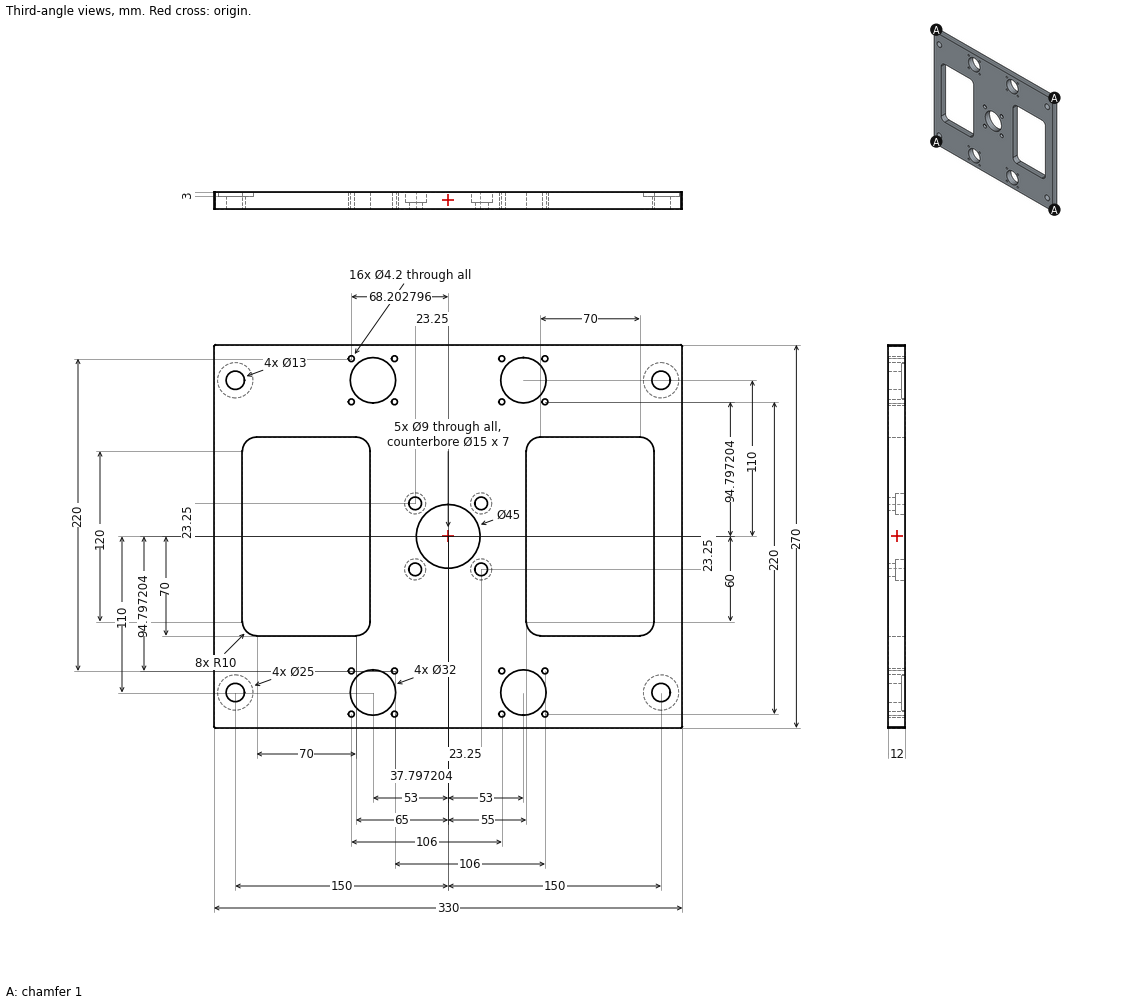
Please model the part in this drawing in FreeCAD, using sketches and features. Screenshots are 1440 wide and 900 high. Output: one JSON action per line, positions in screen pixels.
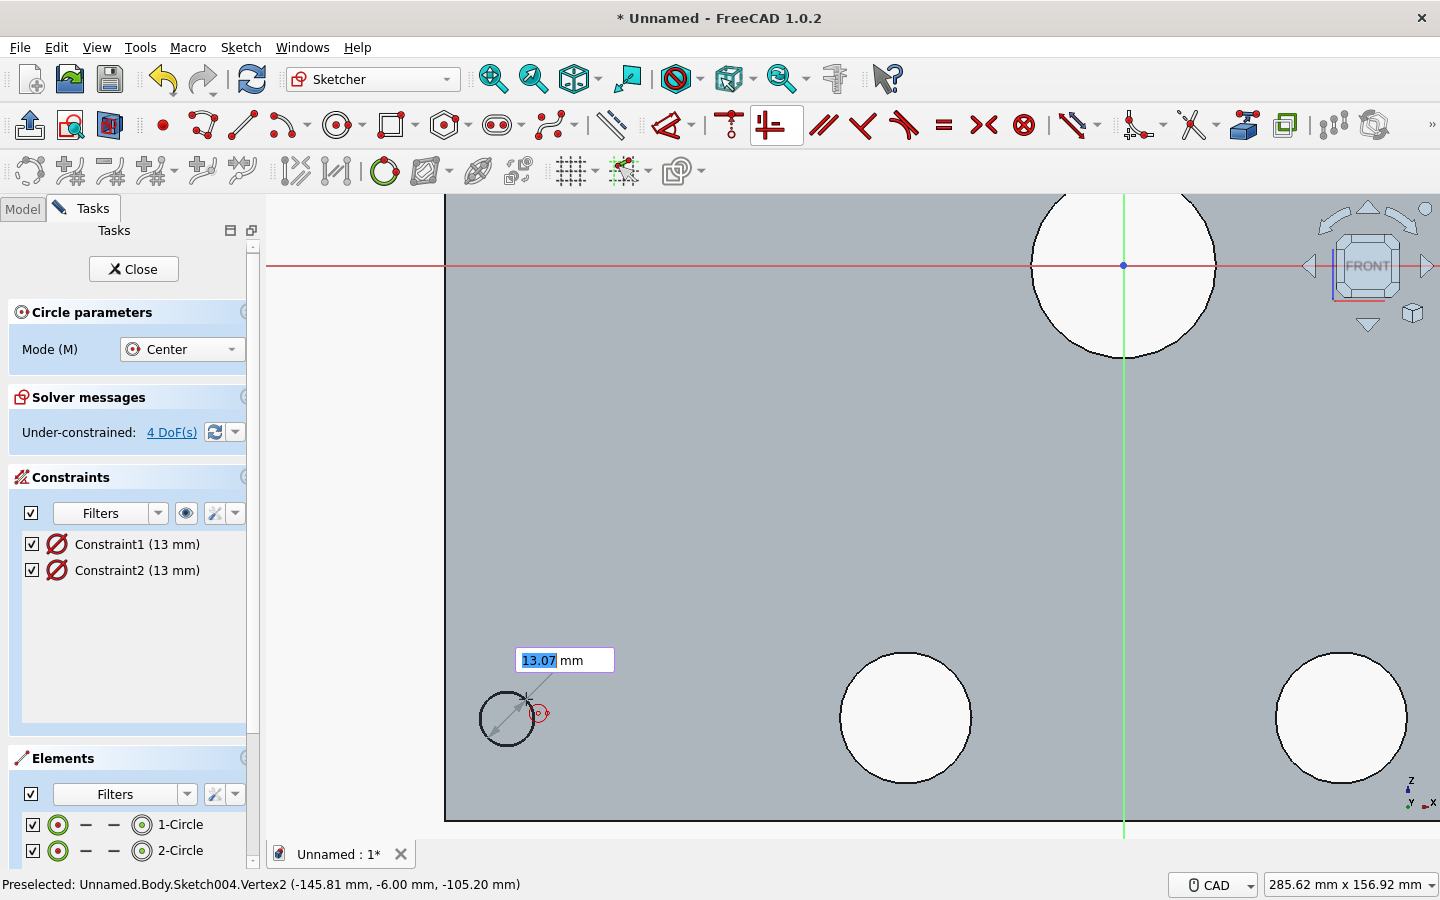
{"action": "type", "text": "13"}
{"action": "key", "text": "Return"}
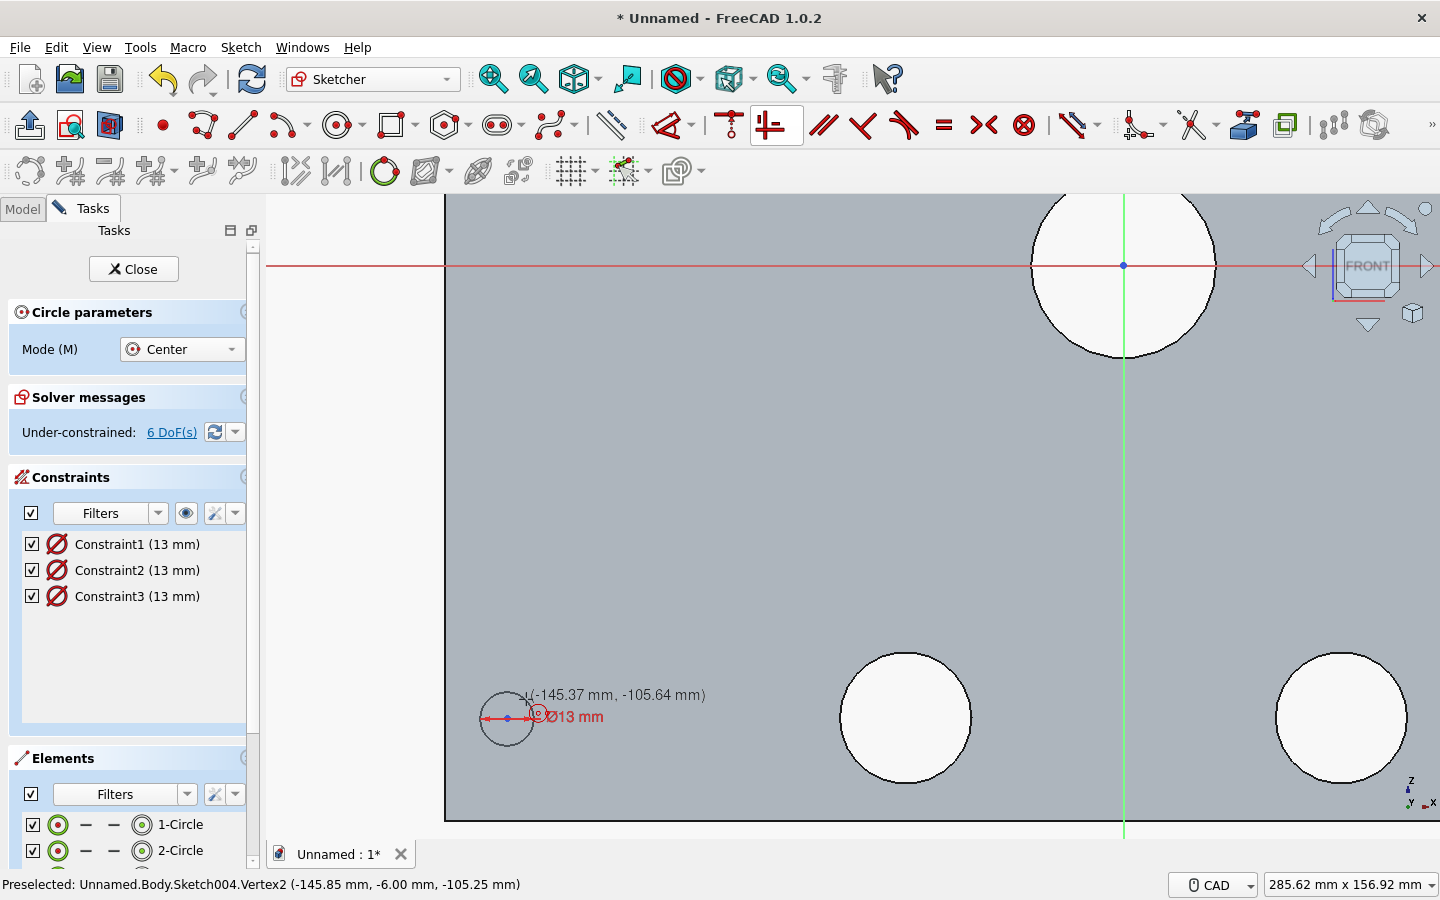
{"action": "scroll", "coordinate": [508, 721], "scroll_direction": "down", "scroll_amount": 4}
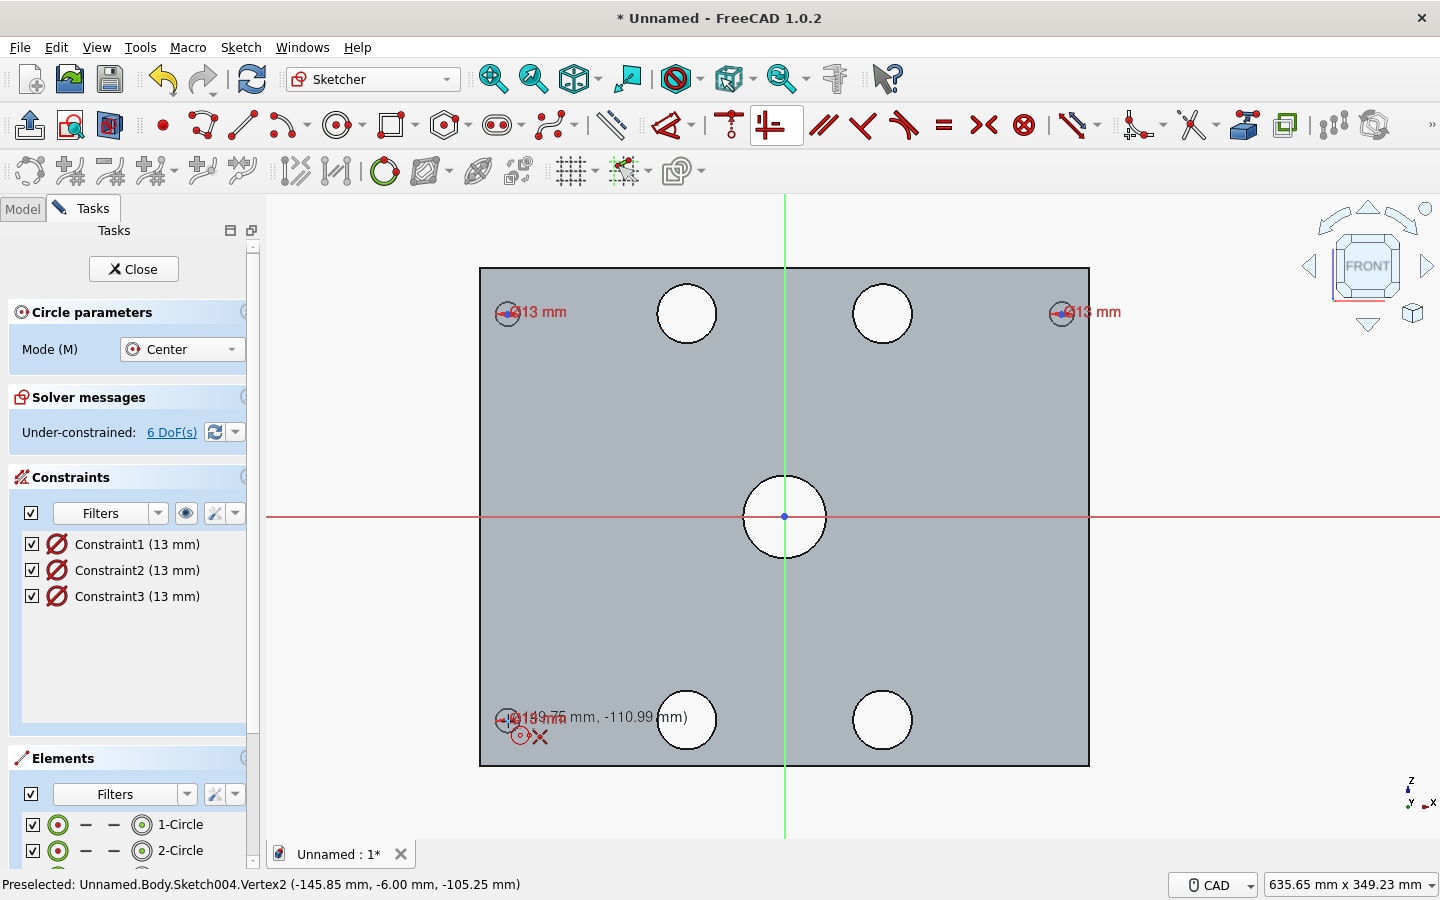
{"action": "scroll", "coordinate": [1062, 720], "scroll_direction": "up", "scroll_amount": 4}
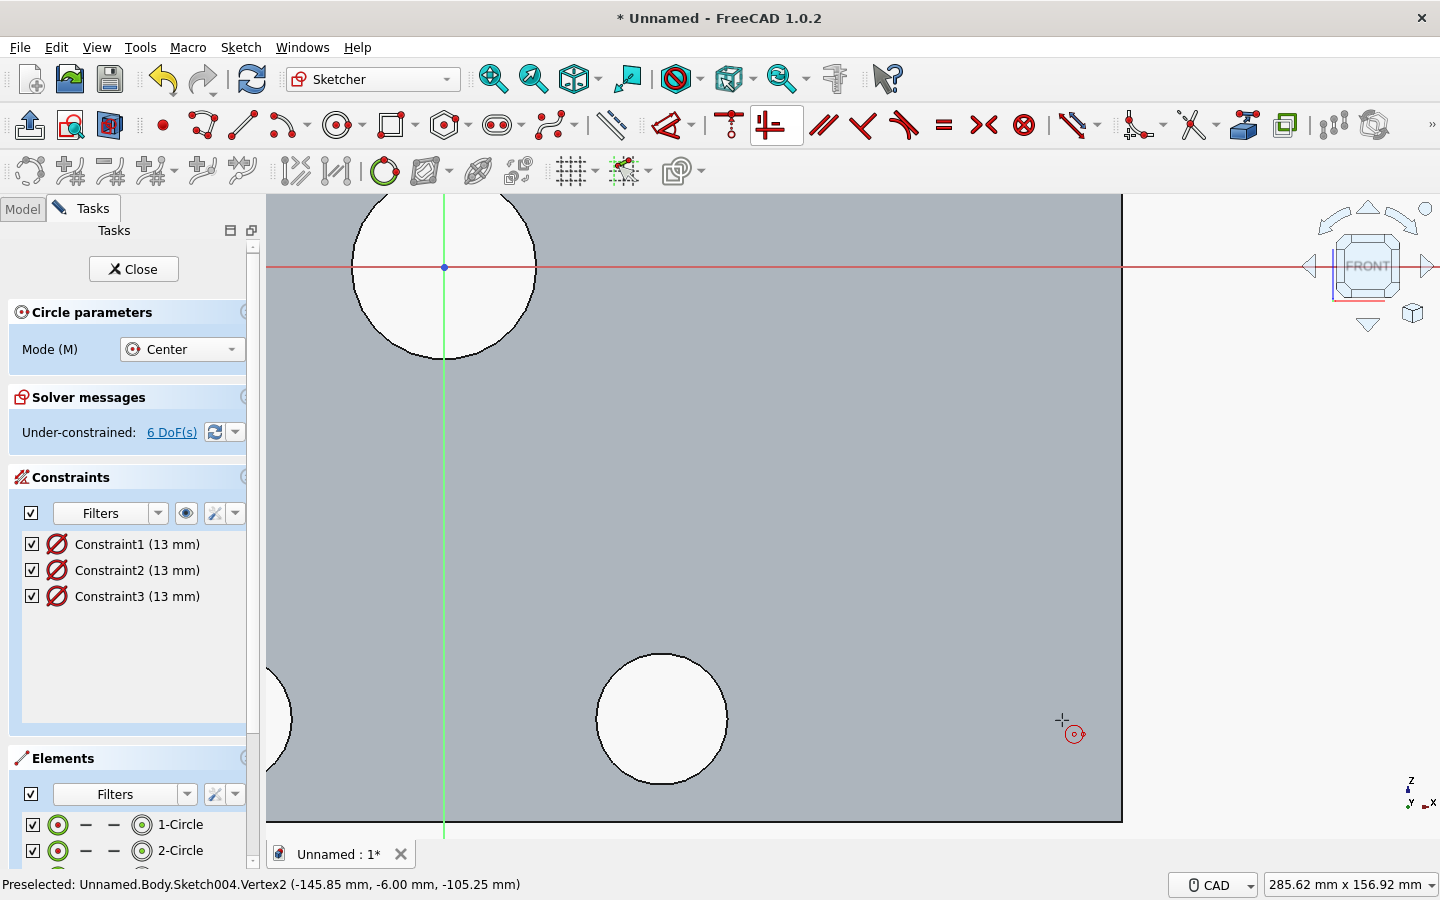
{"action": "left_click", "coordinate": [1061, 719]}
{"action": "mouse_move", "coordinate": [1079, 700]}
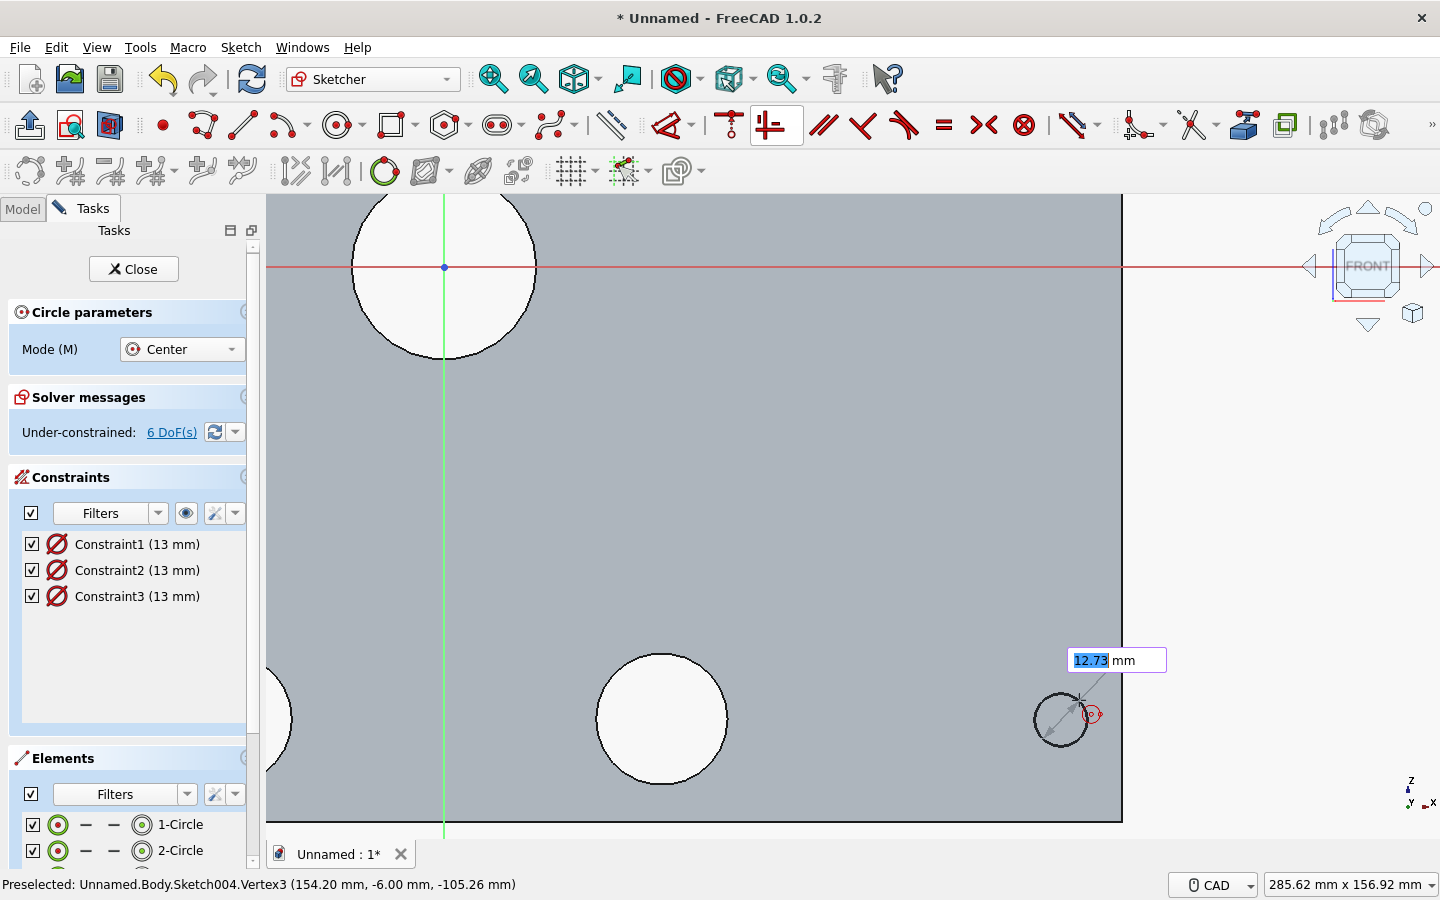
{"action": "type", "text": "13"}
{"action": "key", "text": "Return"}
{"action": "key", "text": "Escape"}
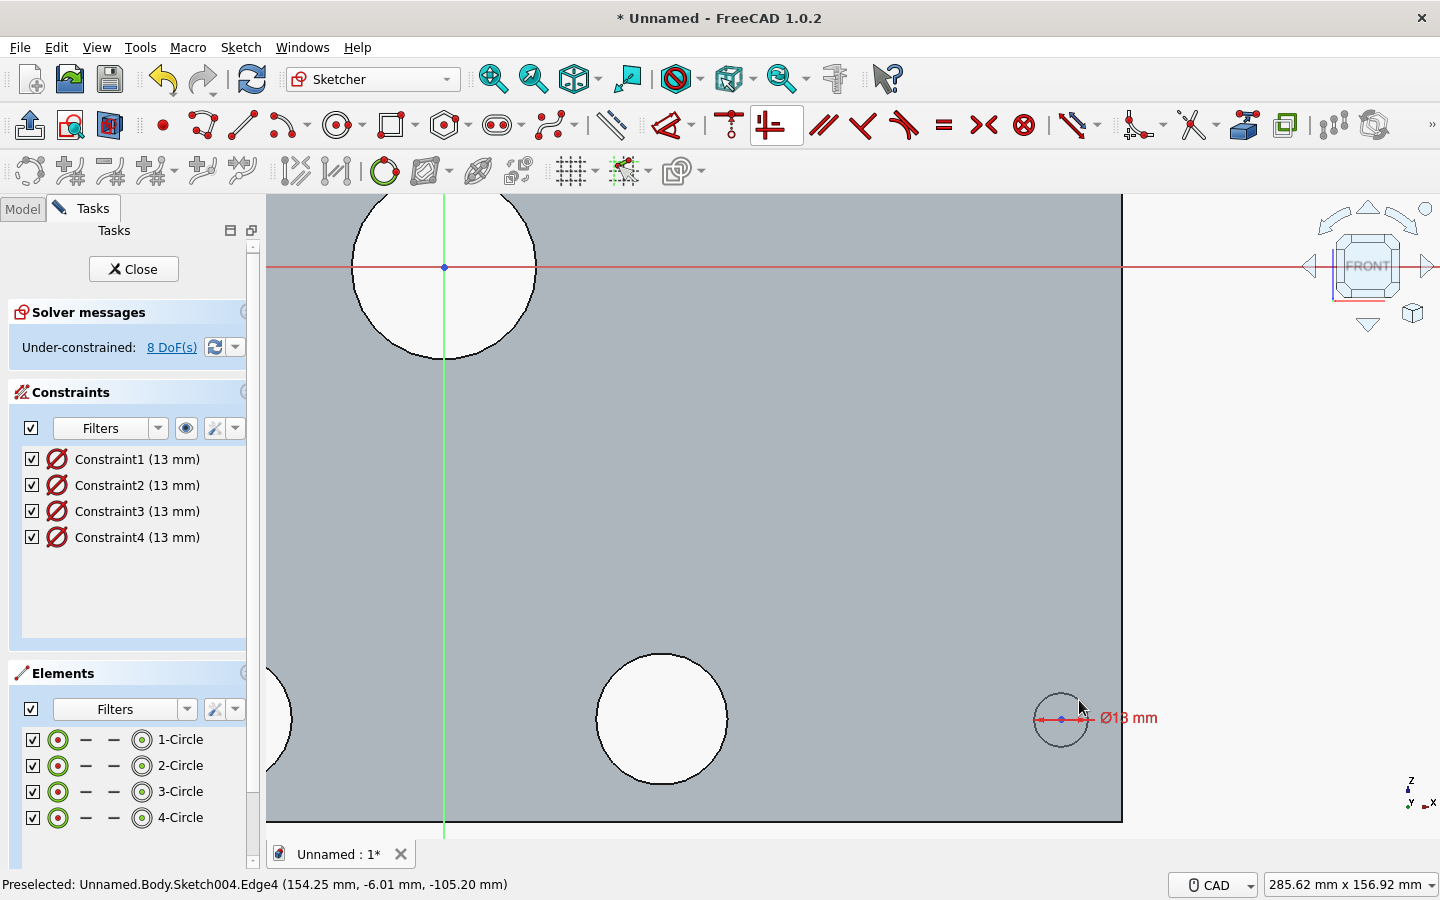
{"action": "scroll", "coordinate": [1062, 720], "scroll_direction": "down", "scroll_amount": 4}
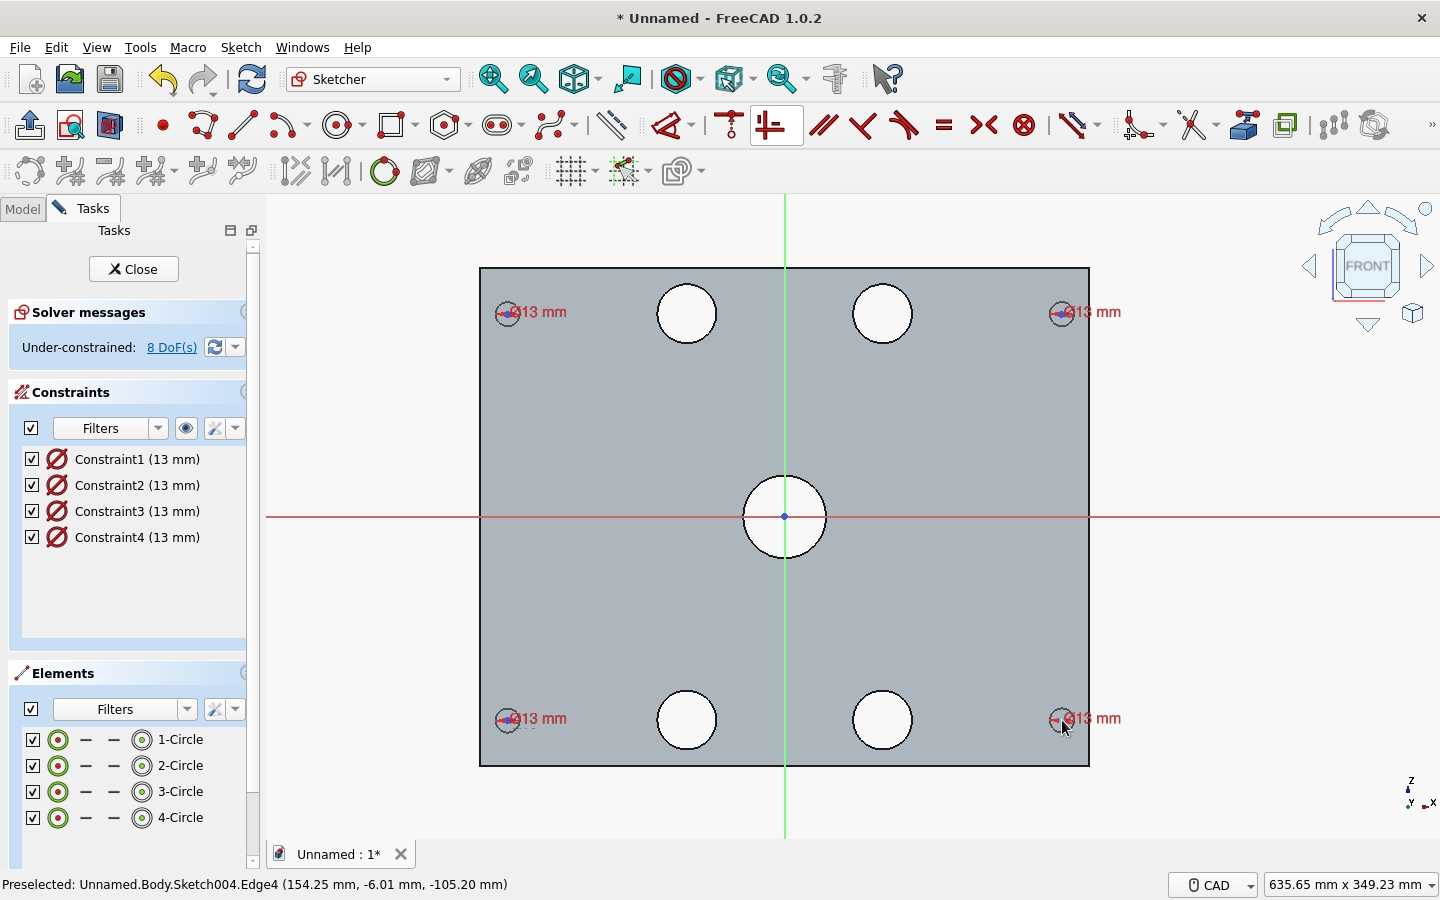
{"action": "left_click", "coordinate": [508, 314]}